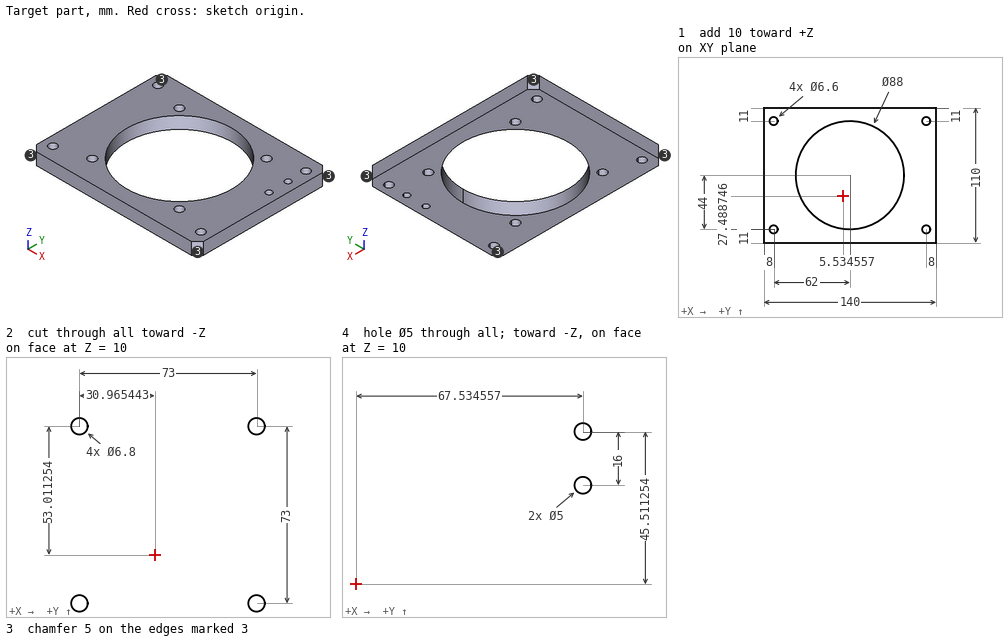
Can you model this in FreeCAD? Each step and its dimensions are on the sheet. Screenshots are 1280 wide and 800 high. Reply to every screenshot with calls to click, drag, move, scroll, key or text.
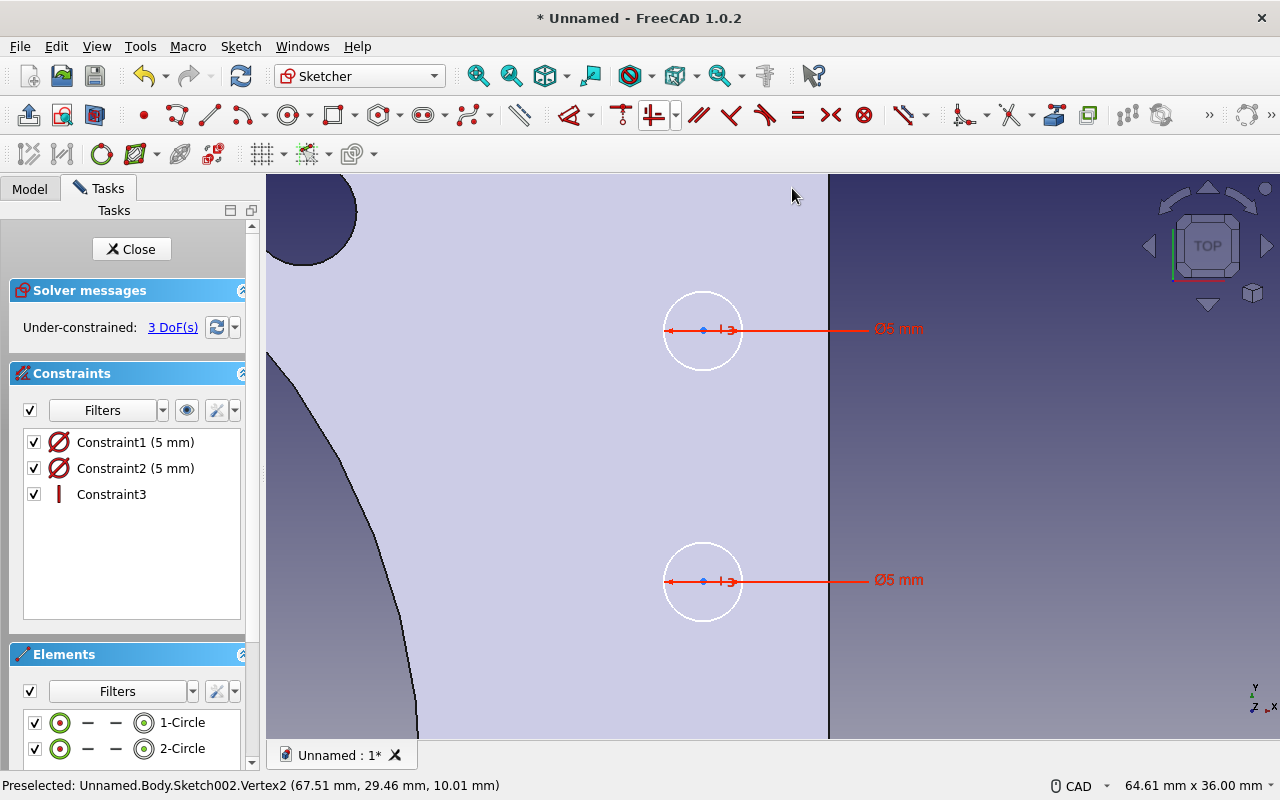
click(568, 116)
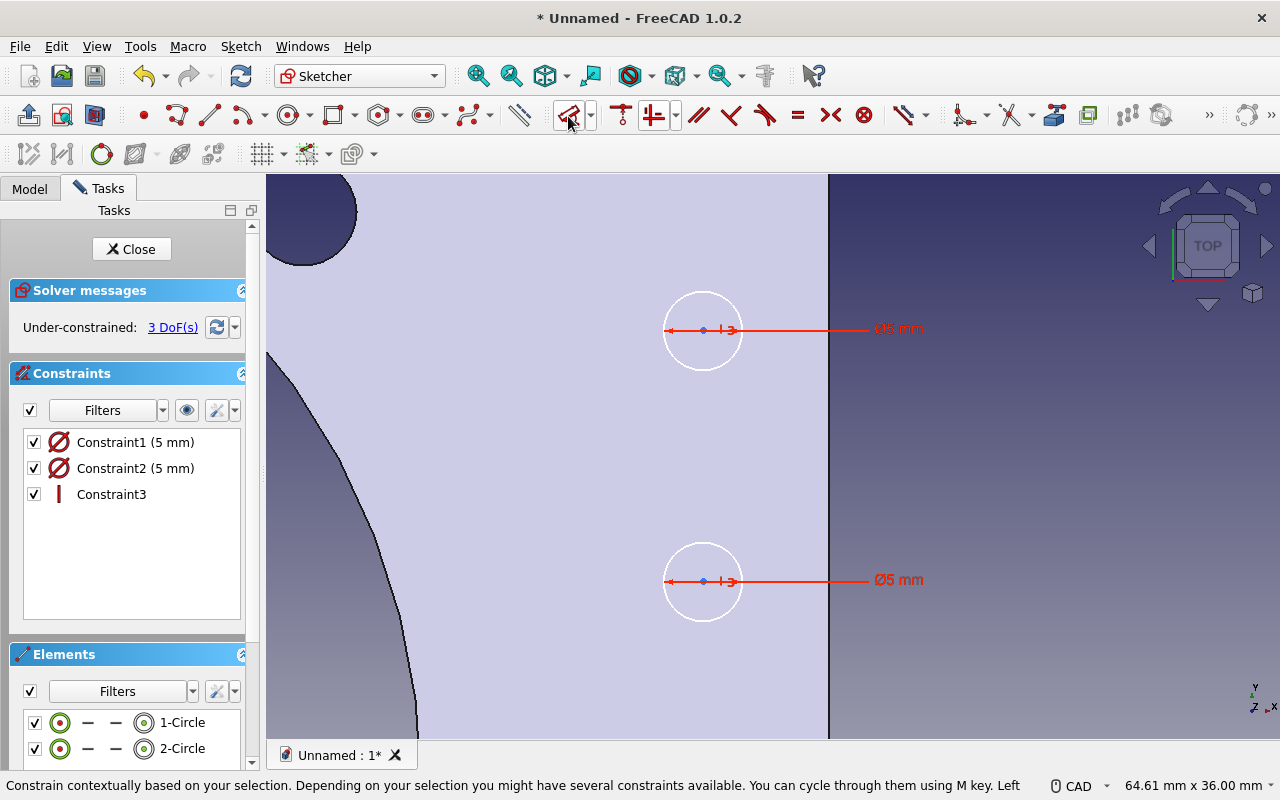
click(703, 331)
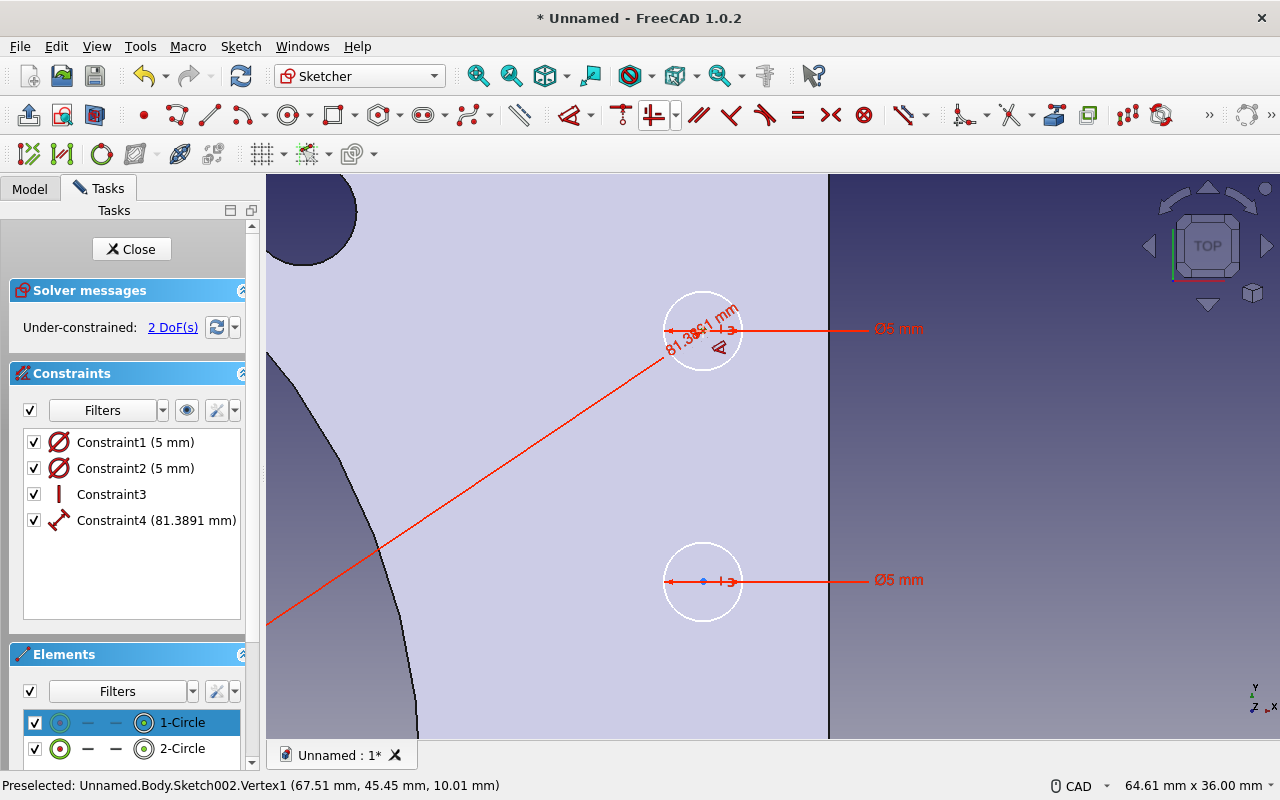
click(703, 582)
click(669, 457)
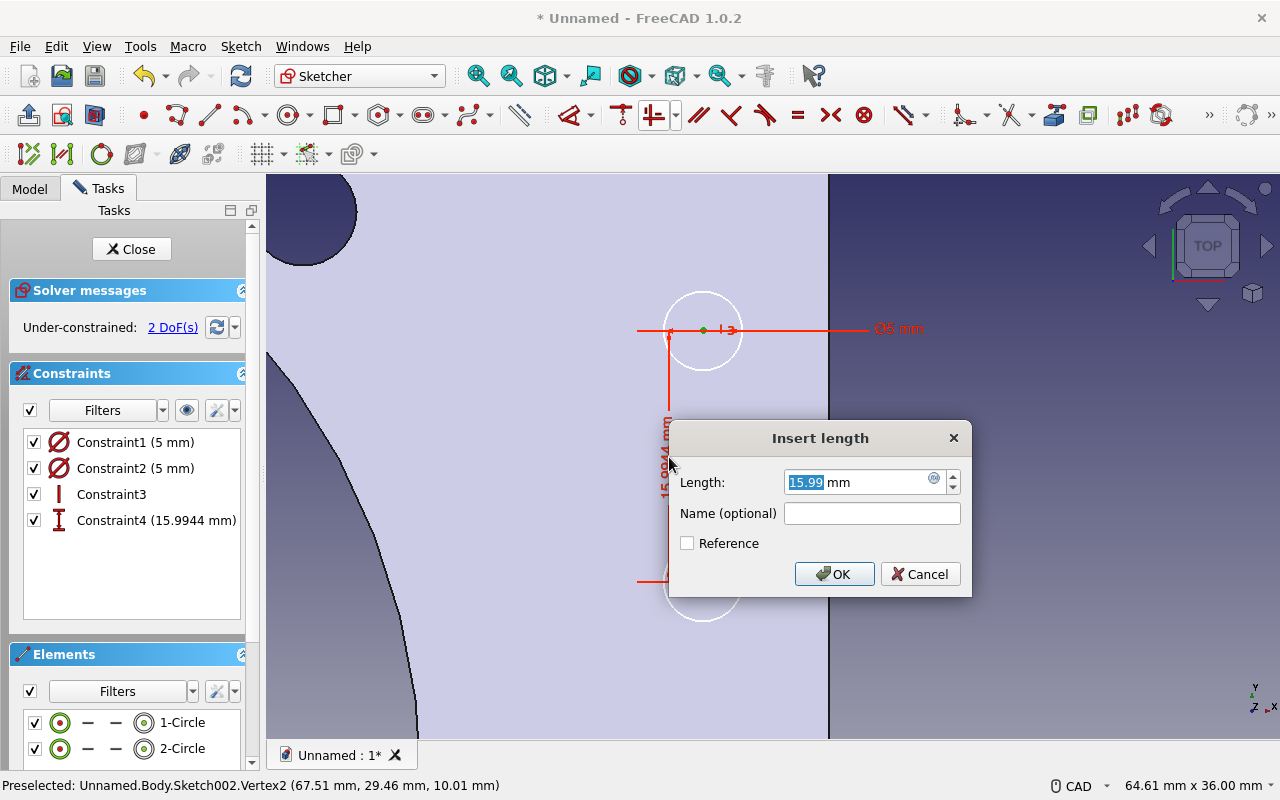
text(16)
key(Return)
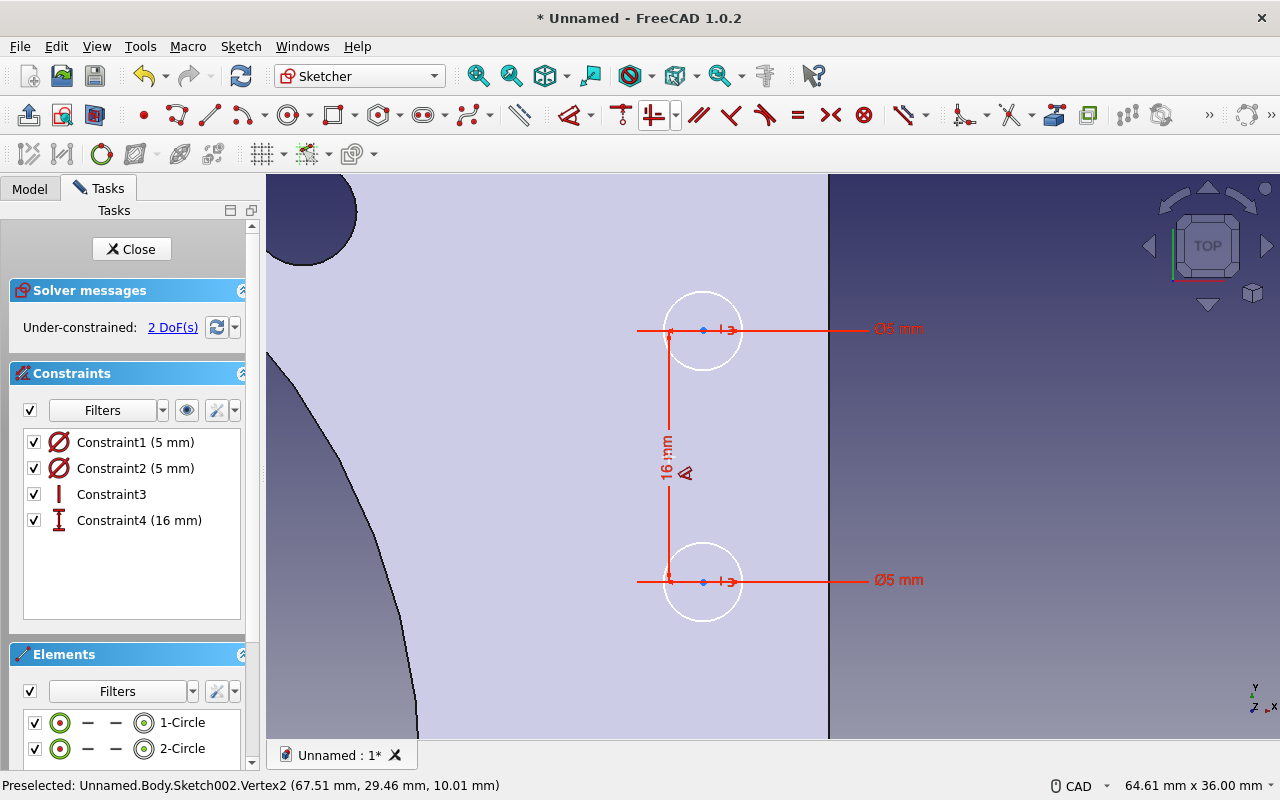
click(703, 331)
click(499, 297)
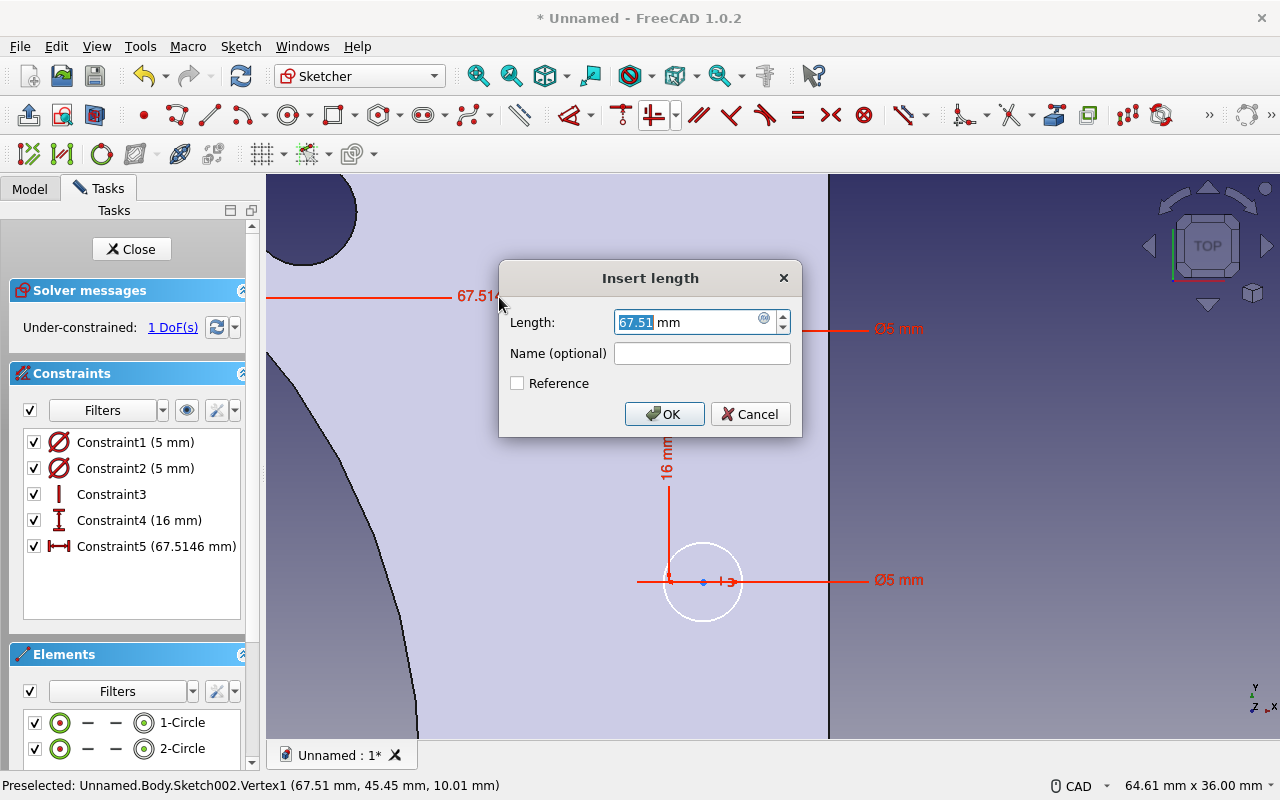
text(67.534557)
key(Return)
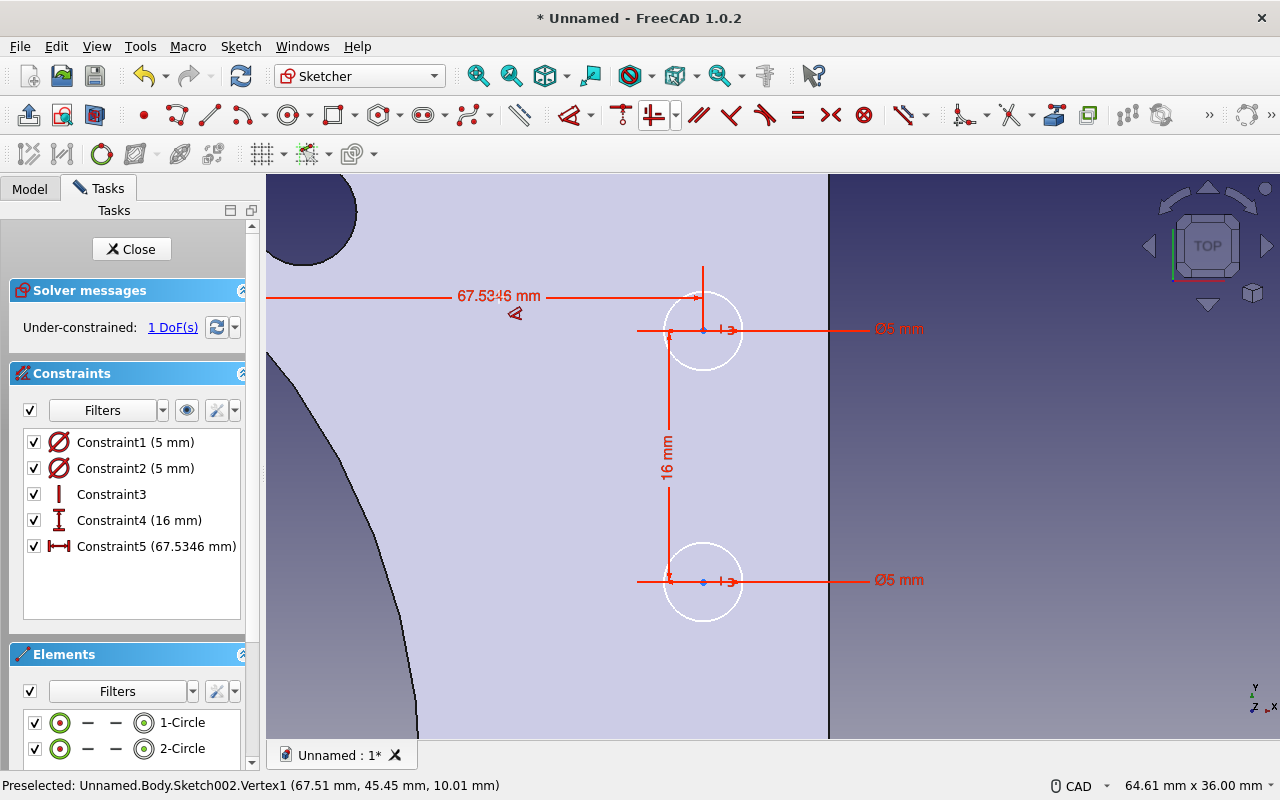
click(703, 331)
click(737, 521)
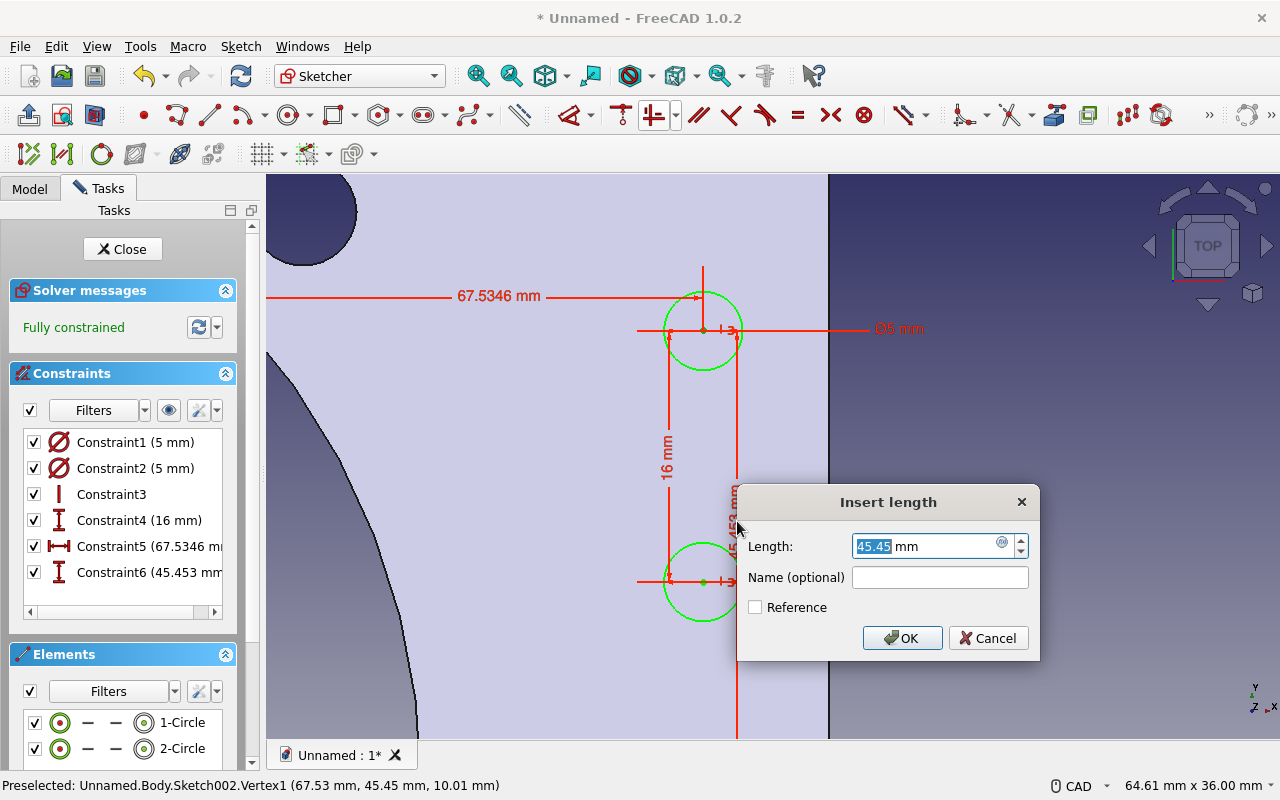
text(45.511254)
key(Return)
key(Escape)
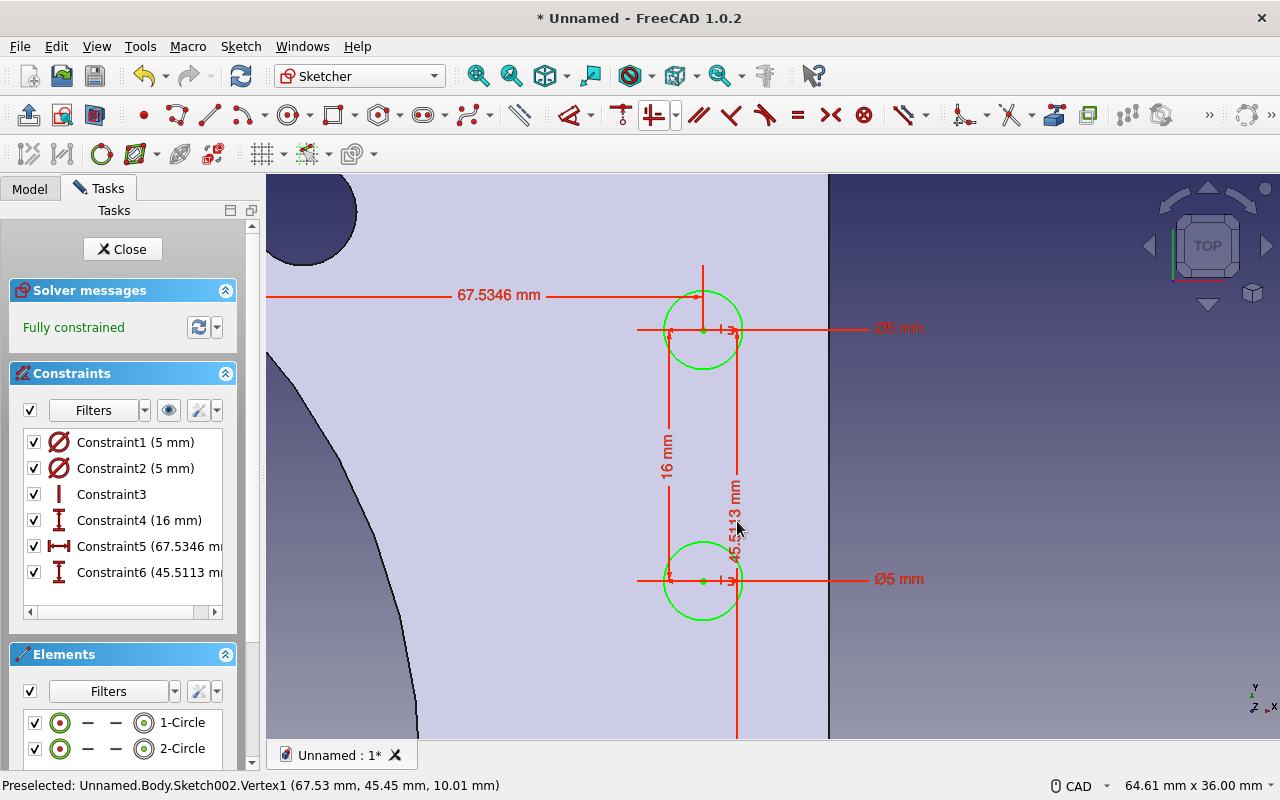
click(123, 249)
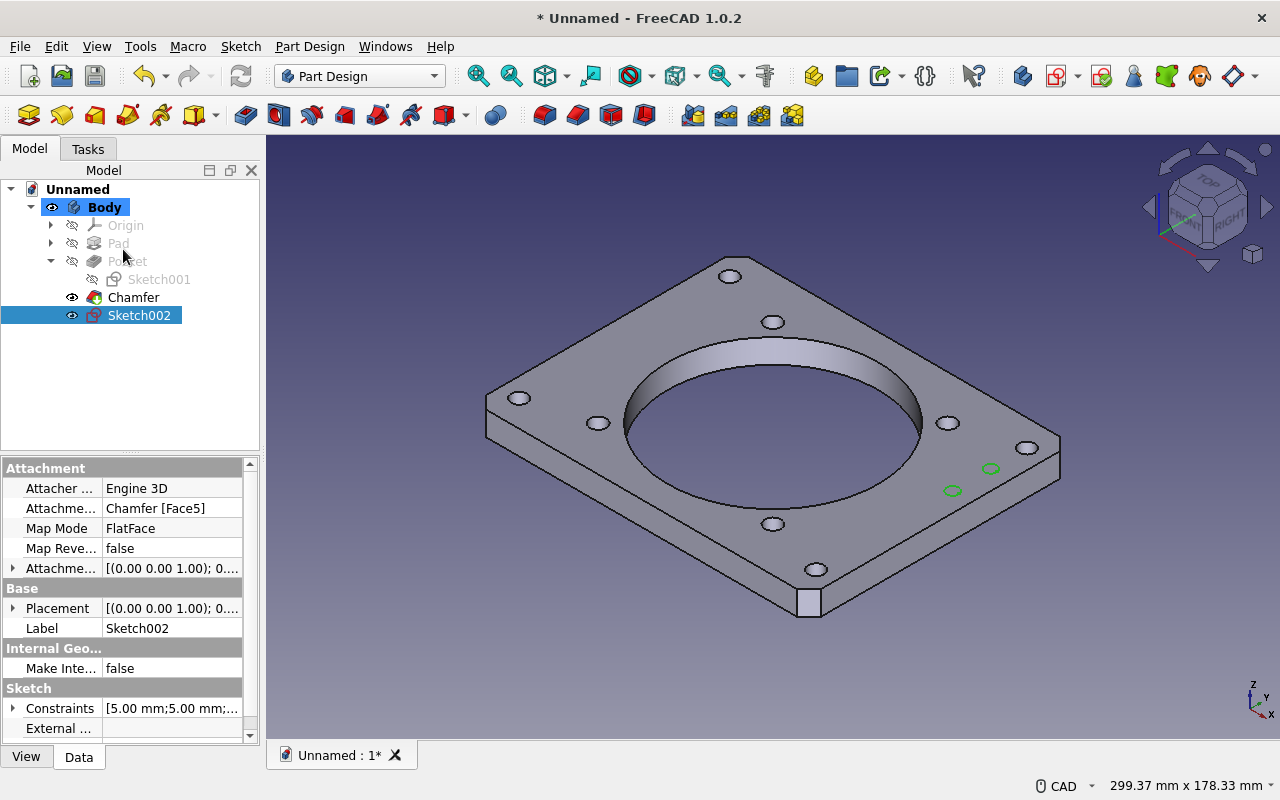
click(279, 116)